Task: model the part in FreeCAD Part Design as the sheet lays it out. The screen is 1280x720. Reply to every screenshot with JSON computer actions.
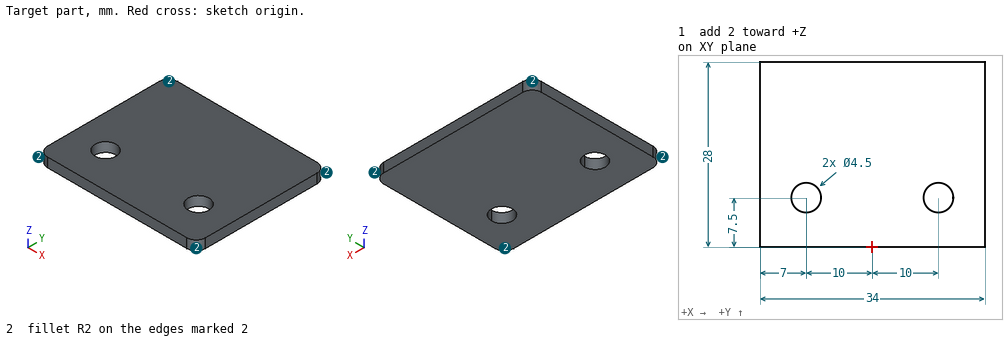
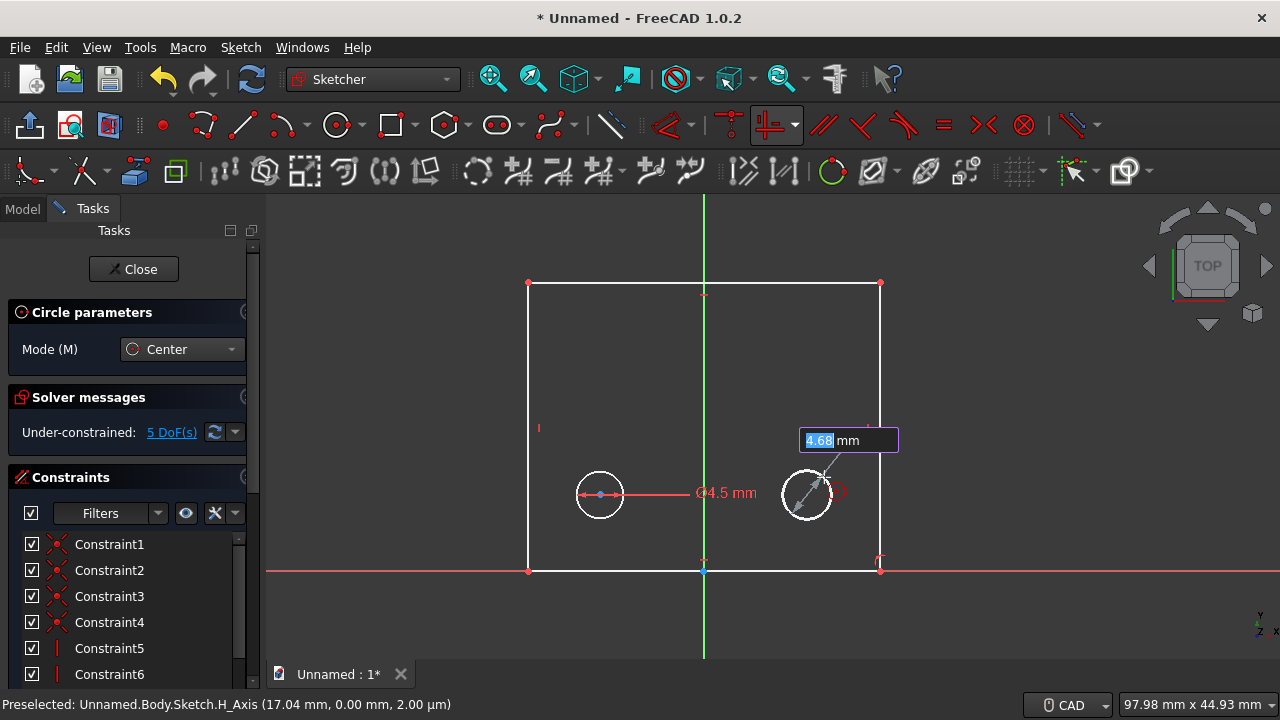
{"action": "type", "text": "4.5"}
{"action": "key", "text": "Return"}
{"action": "key", "text": "Escape"}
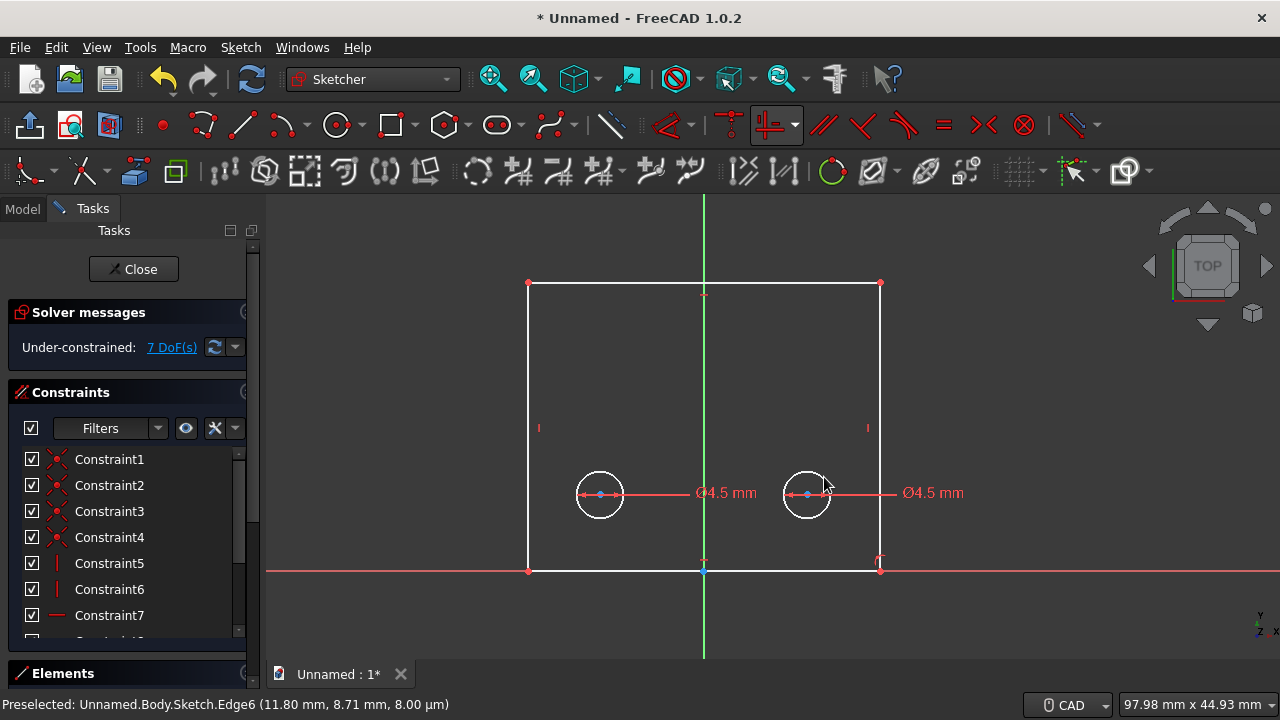
{"action": "left_click", "coordinate": [600, 495]}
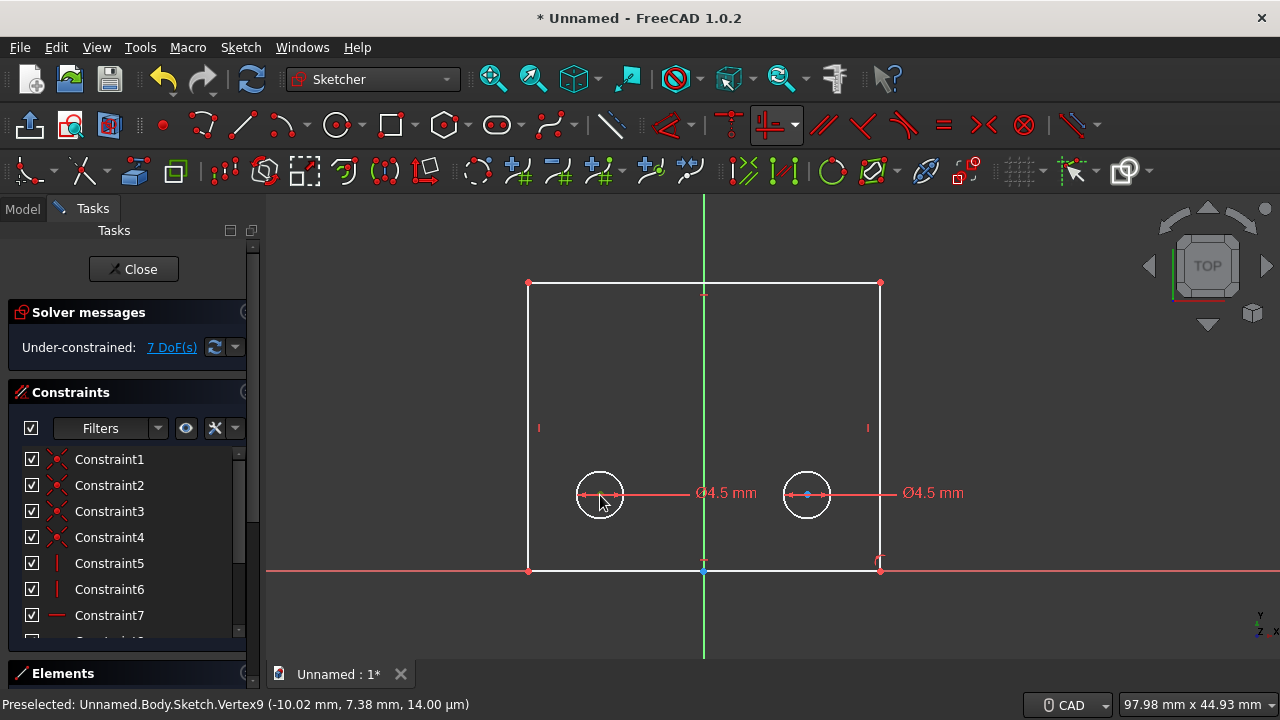
{"action": "left_click", "coordinate": [807, 495]}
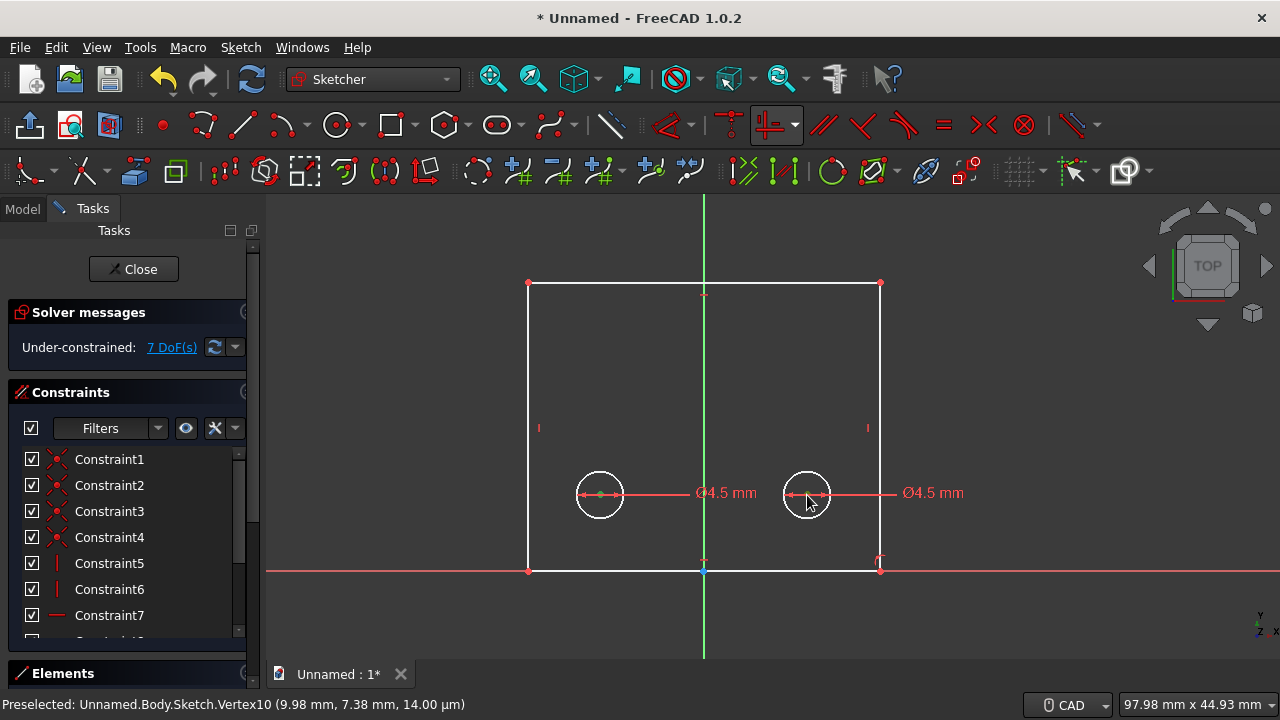
{"action": "key", "text": "h"}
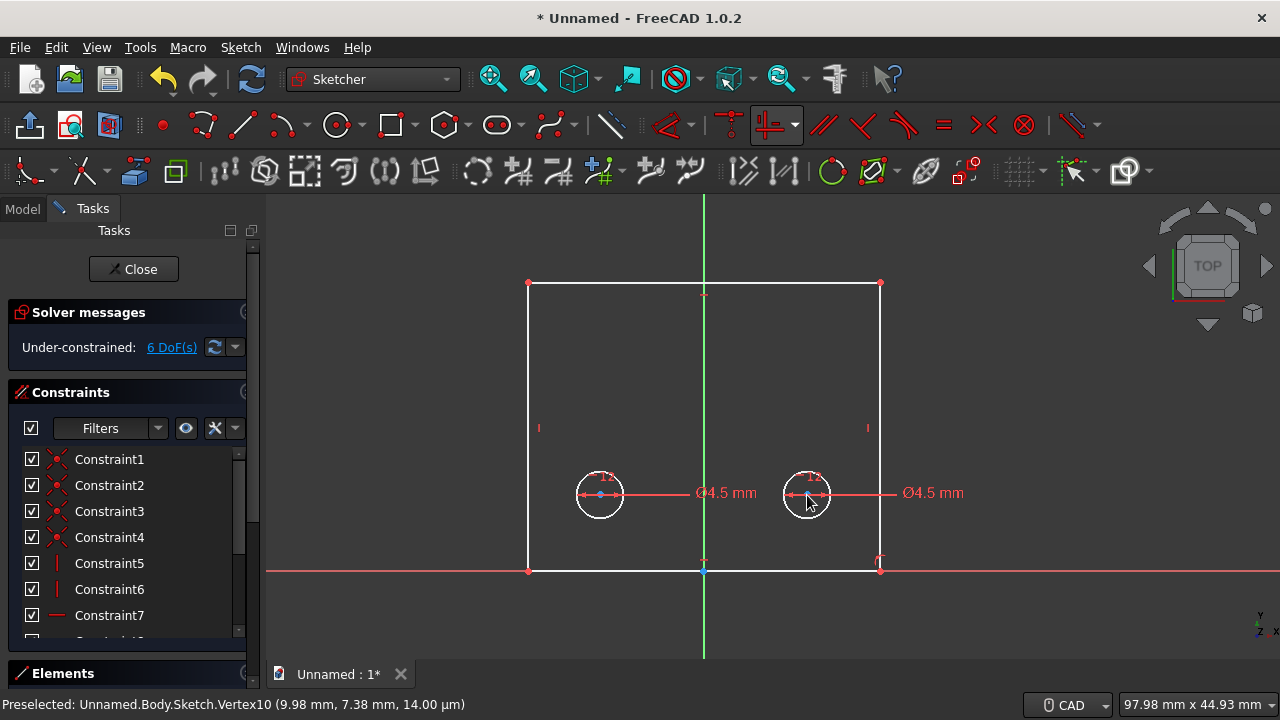
{"action": "left_click", "coordinate": [666, 126]}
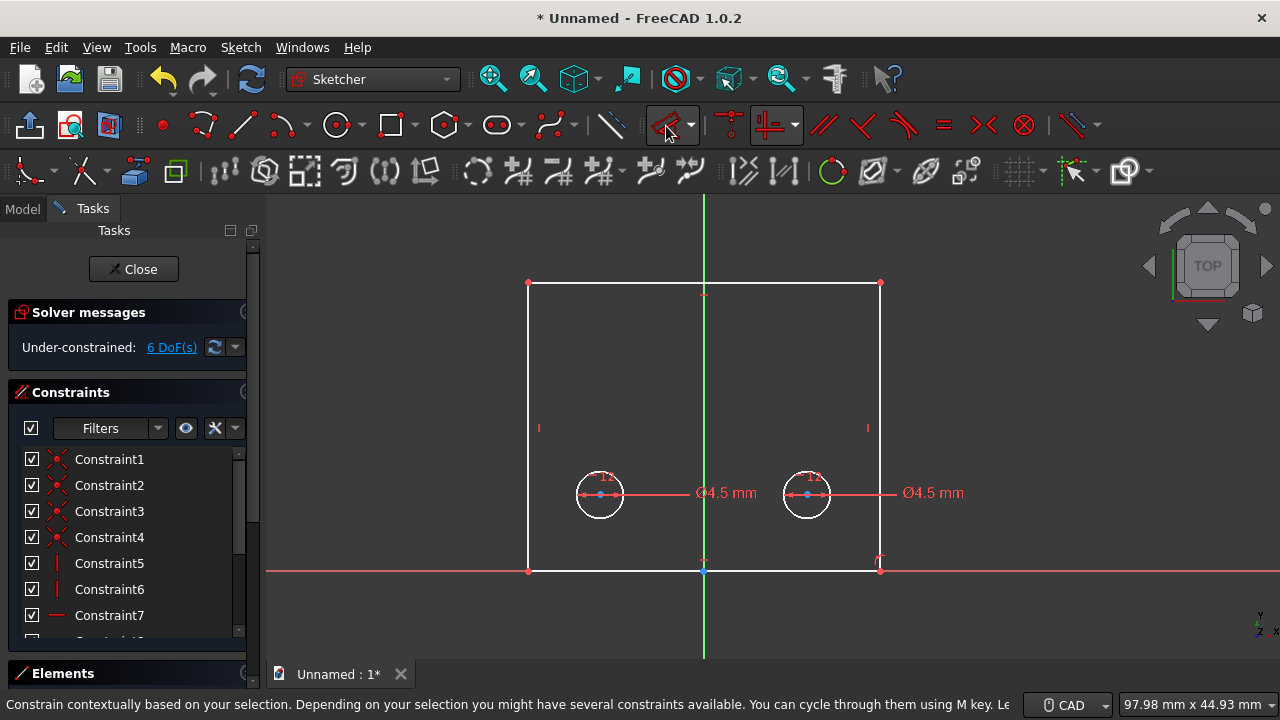
{"action": "left_click", "coordinate": [528, 370]}
{"action": "left_click", "coordinate": [494, 427]}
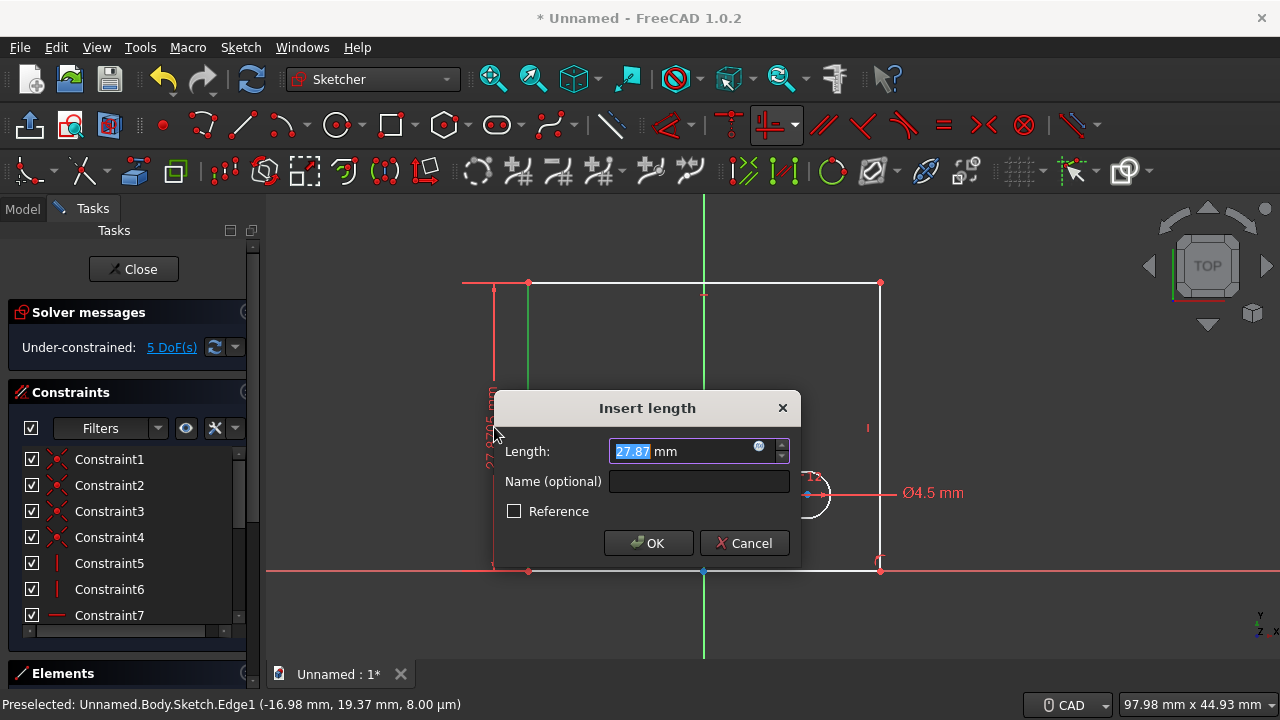
{"action": "type", "text": "28"}
{"action": "key", "text": "Return"}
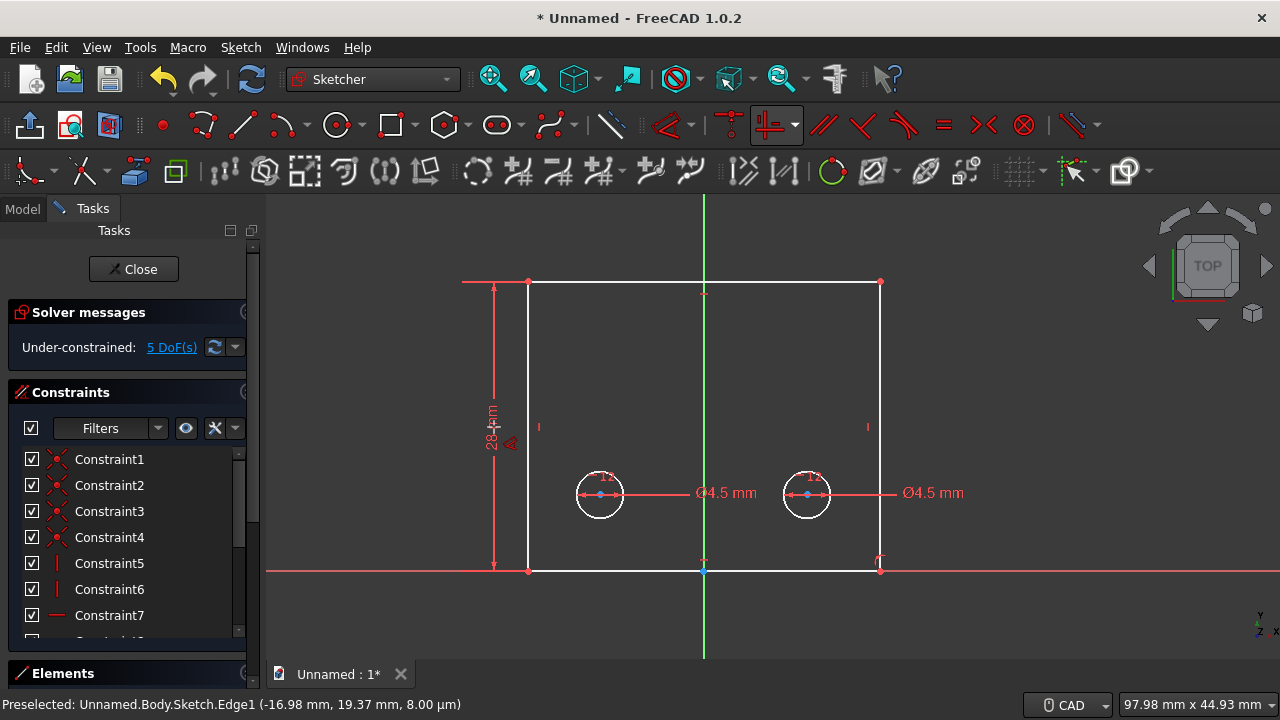
{"action": "left_click", "coordinate": [634, 571]}
{"action": "left_click", "coordinate": [623, 605]}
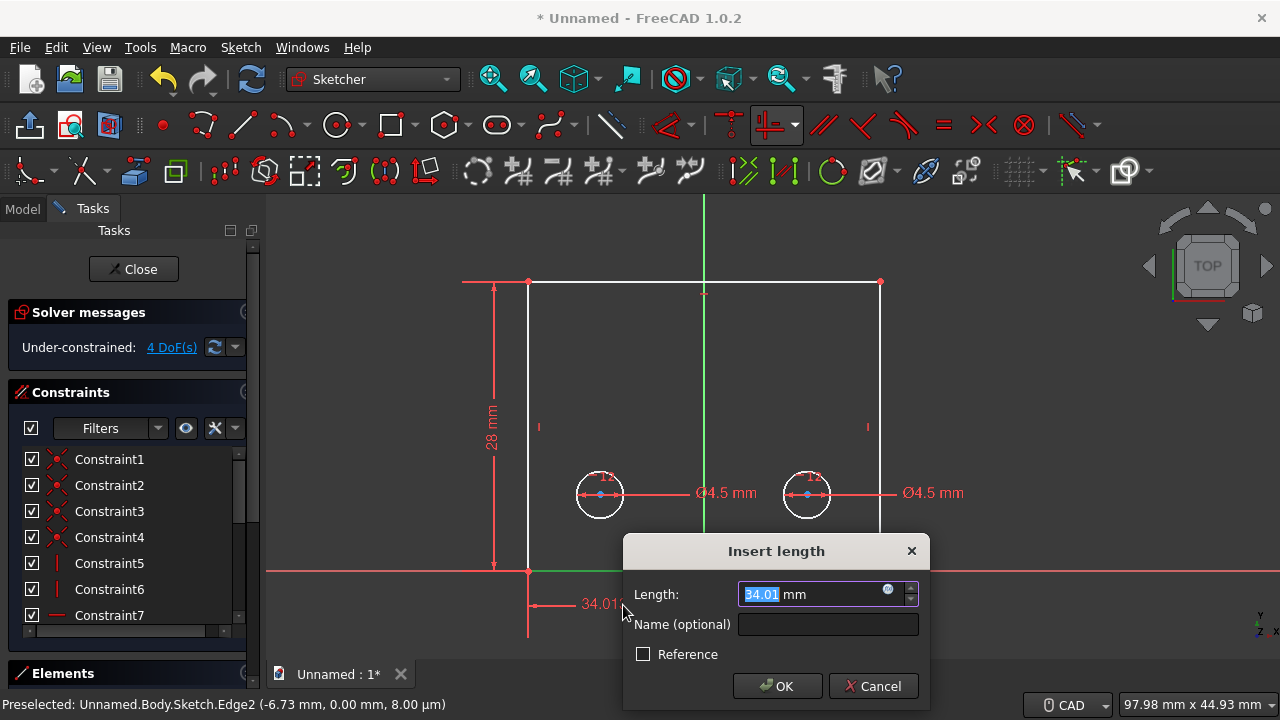
{"action": "type", "text": "34"}
{"action": "key", "text": "Return"}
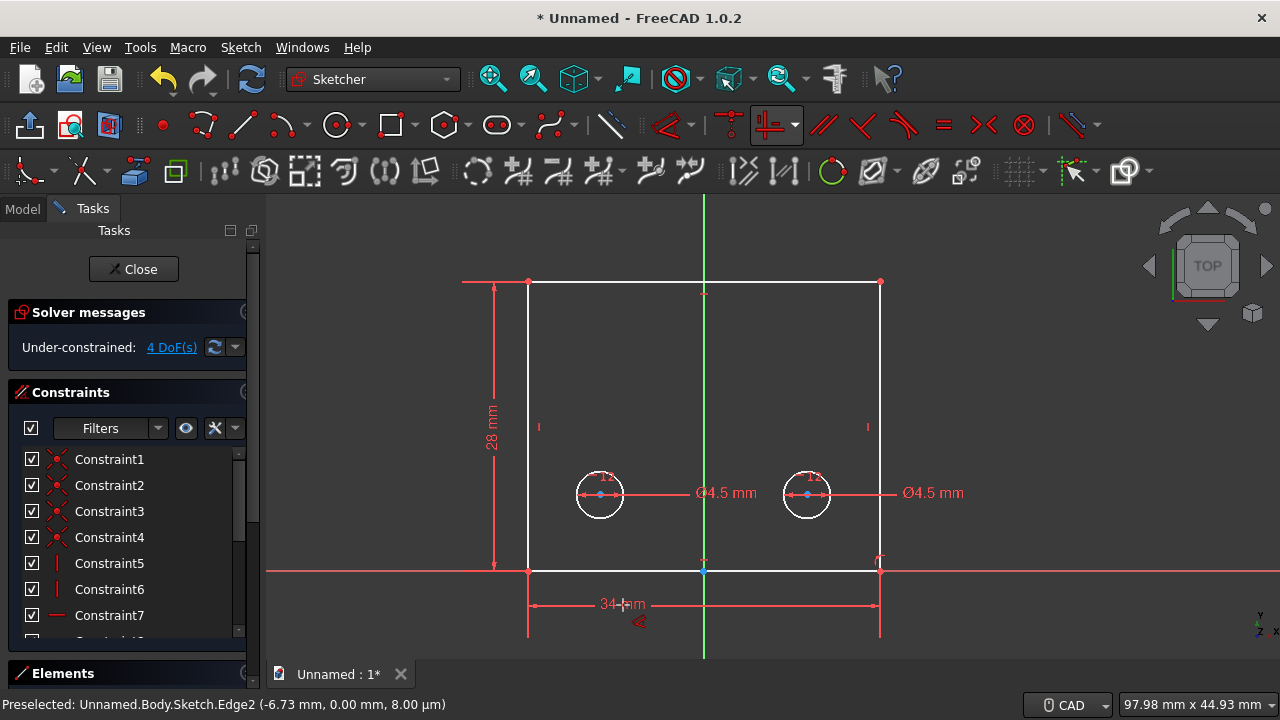
{"action": "left_click", "coordinate": [600, 495]}
{"action": "left_click", "coordinate": [652, 461]}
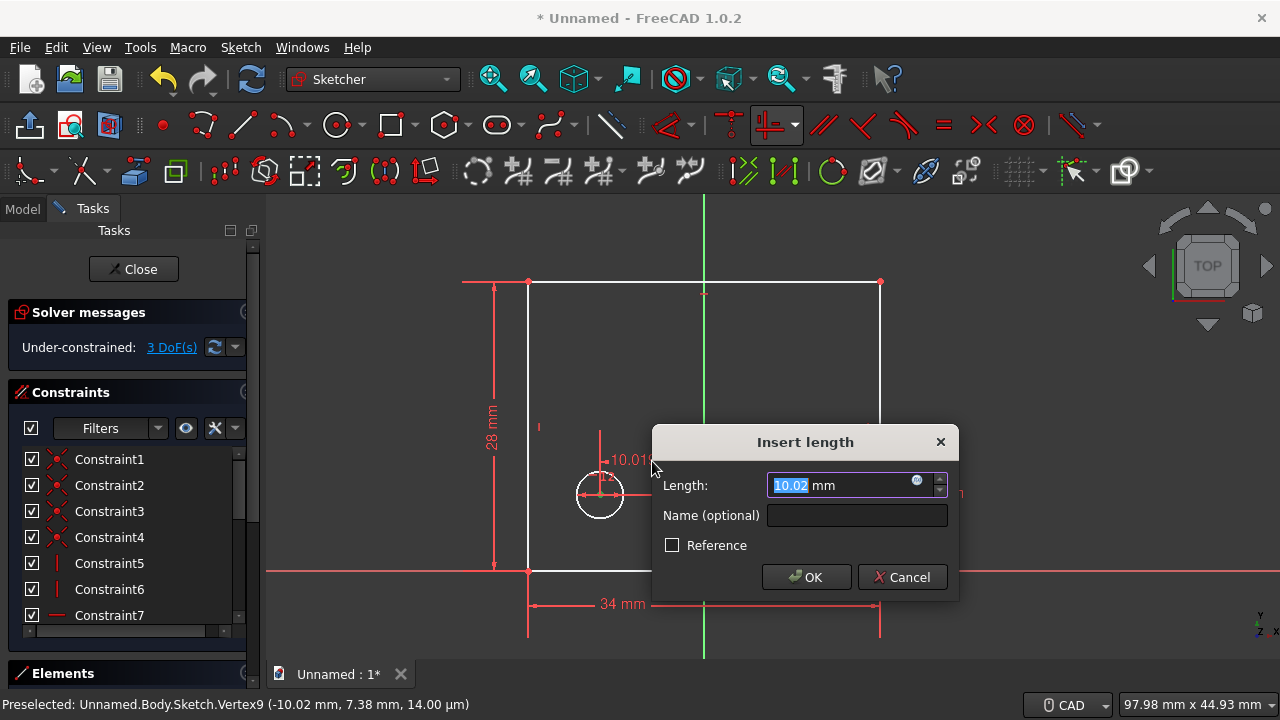
{"action": "type", "text": "10"}
{"action": "key", "text": "Return"}